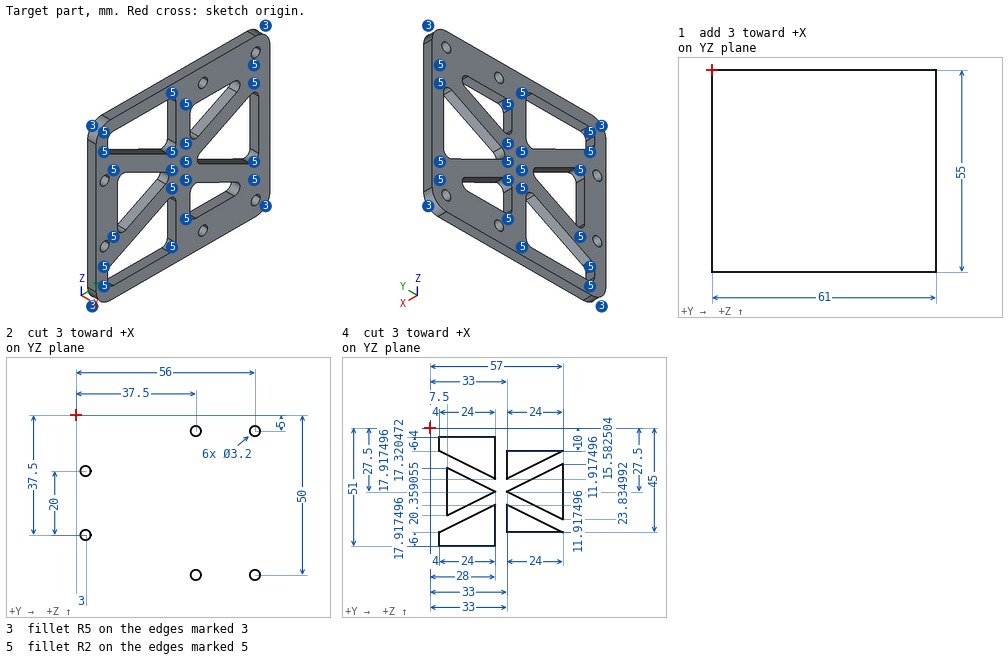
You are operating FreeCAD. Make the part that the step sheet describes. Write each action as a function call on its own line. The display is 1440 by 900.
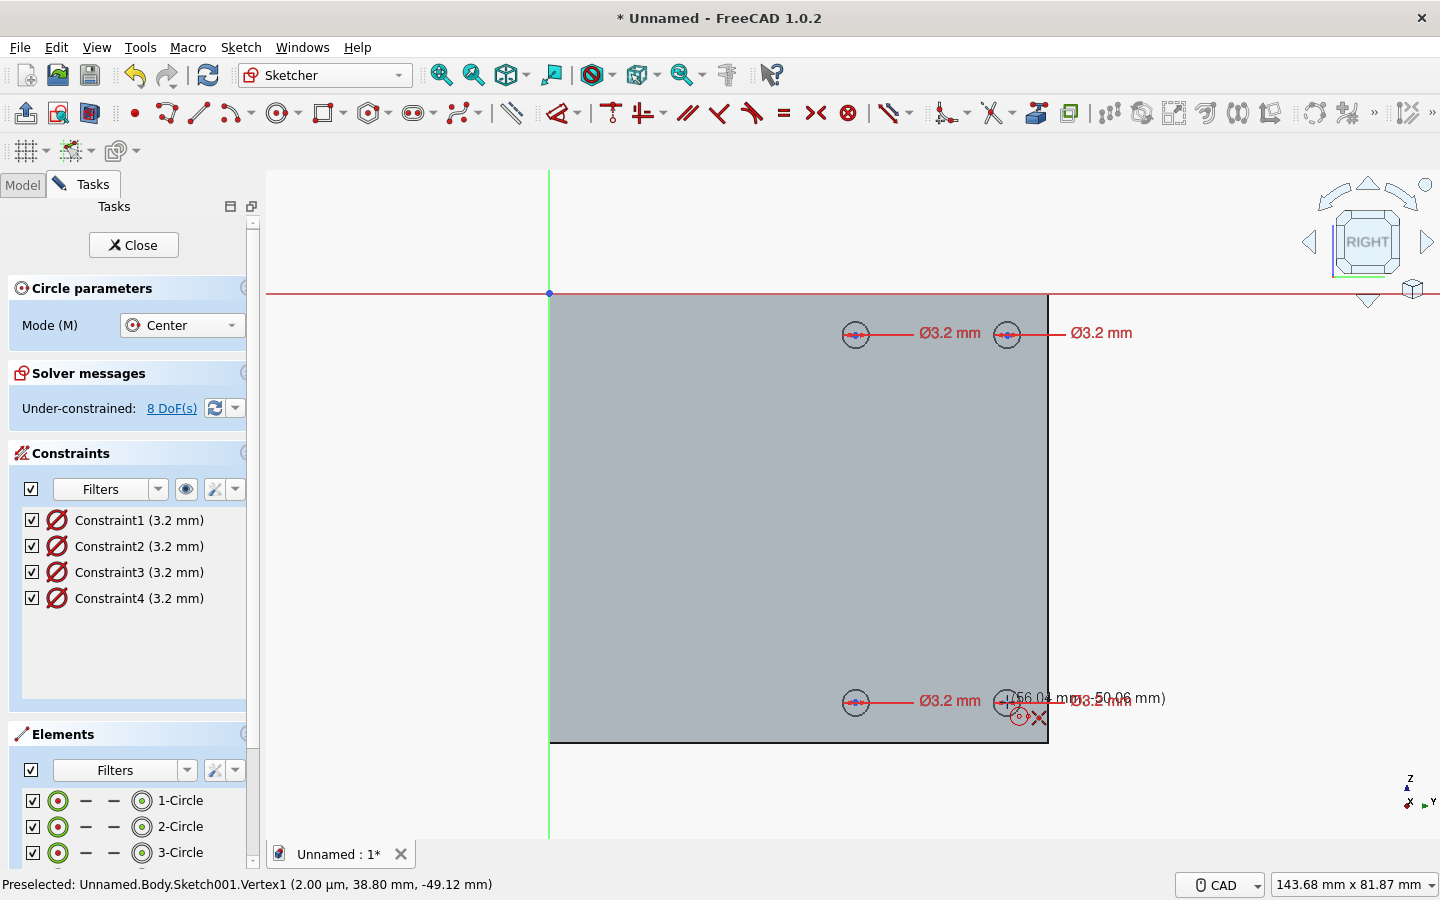
scroll(574, 600, up, 3)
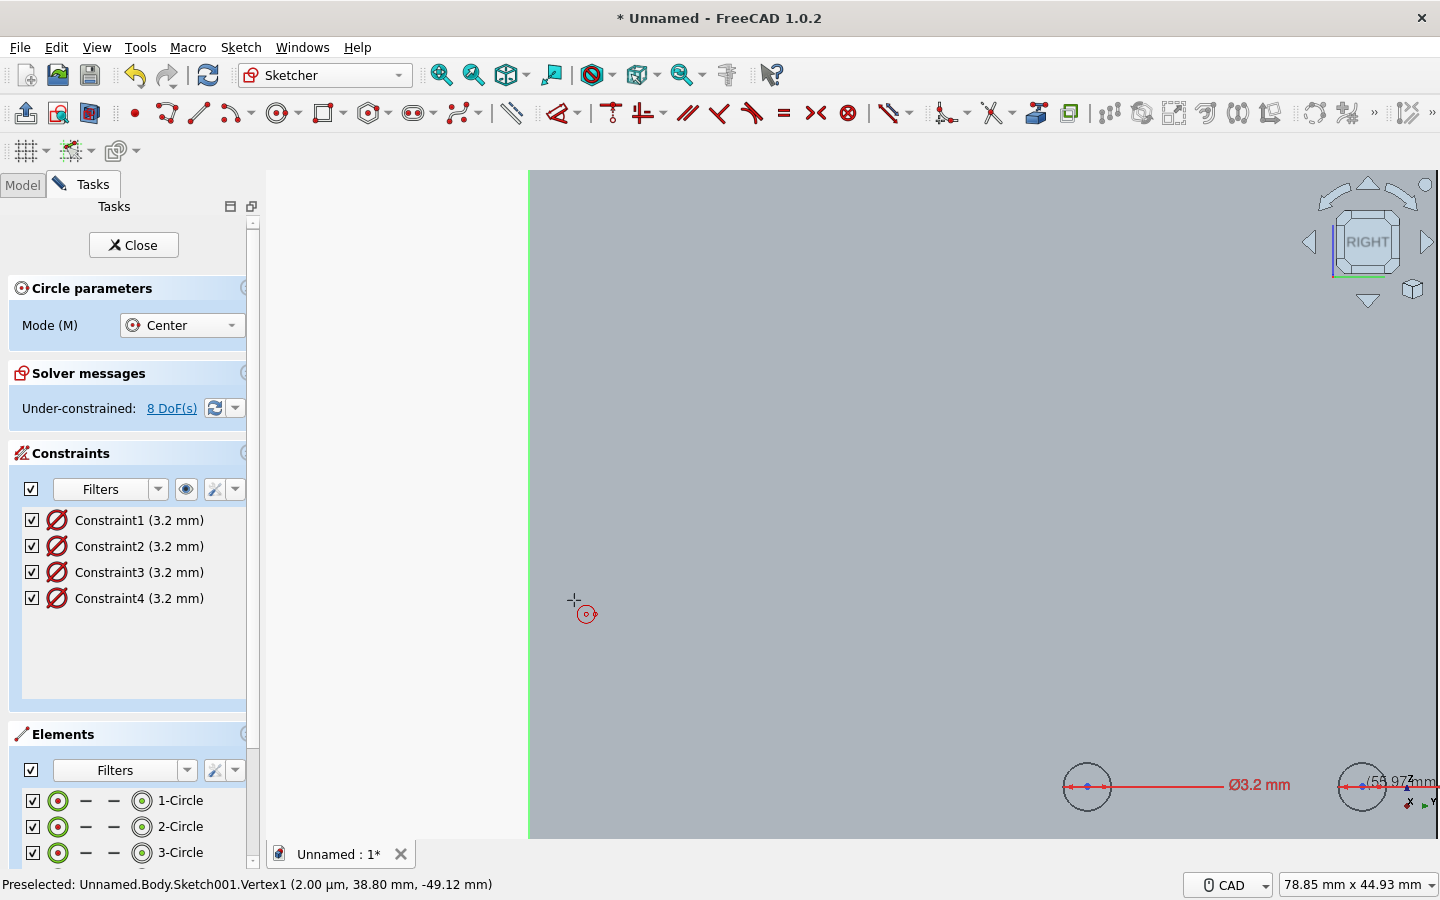
click(574, 600)
move(590, 583)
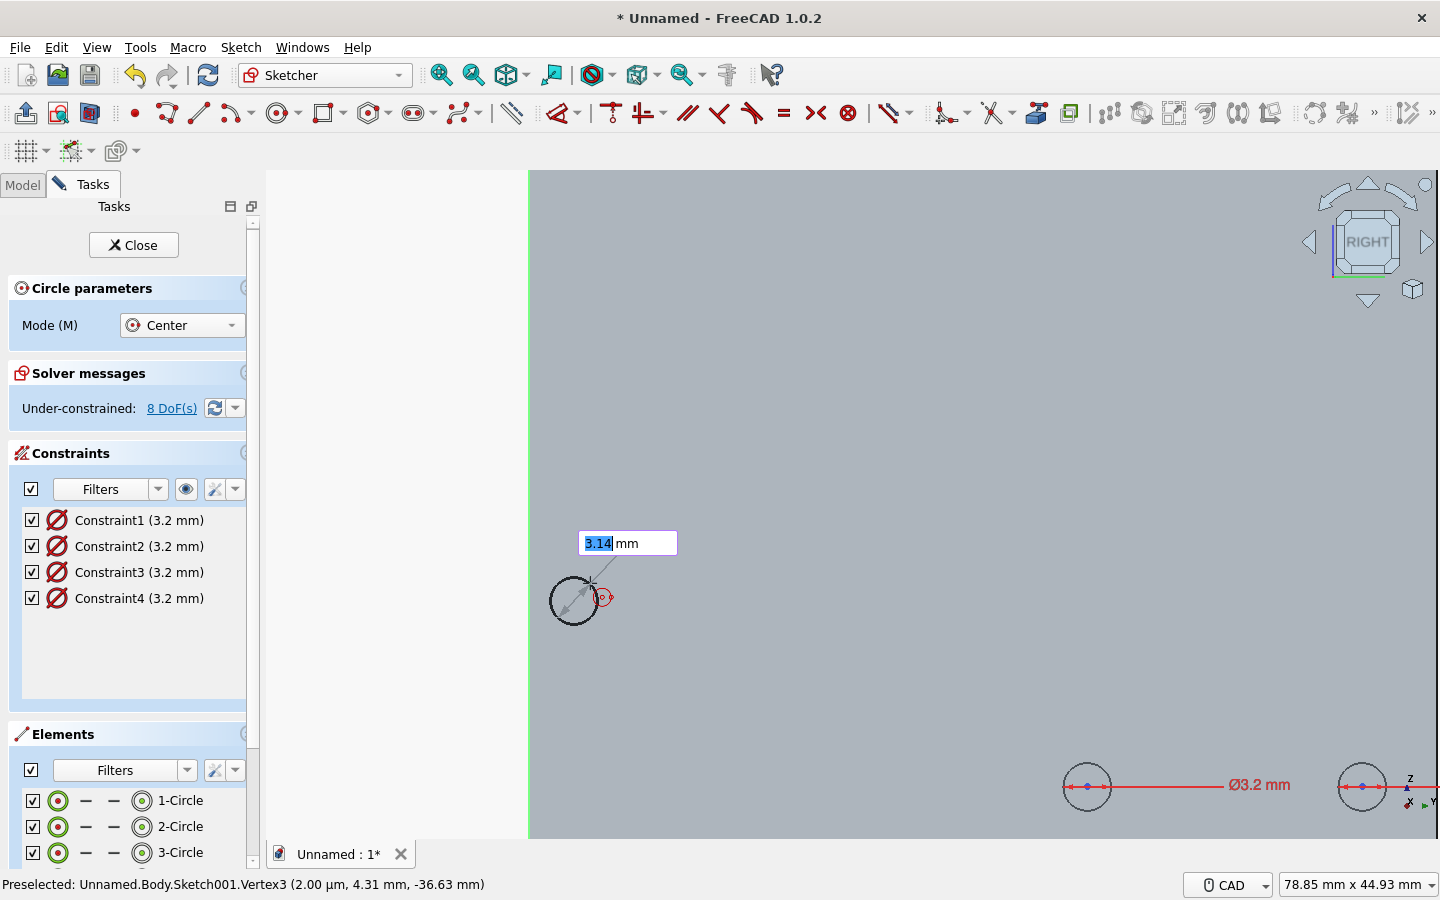
text(3.2)
key(Return)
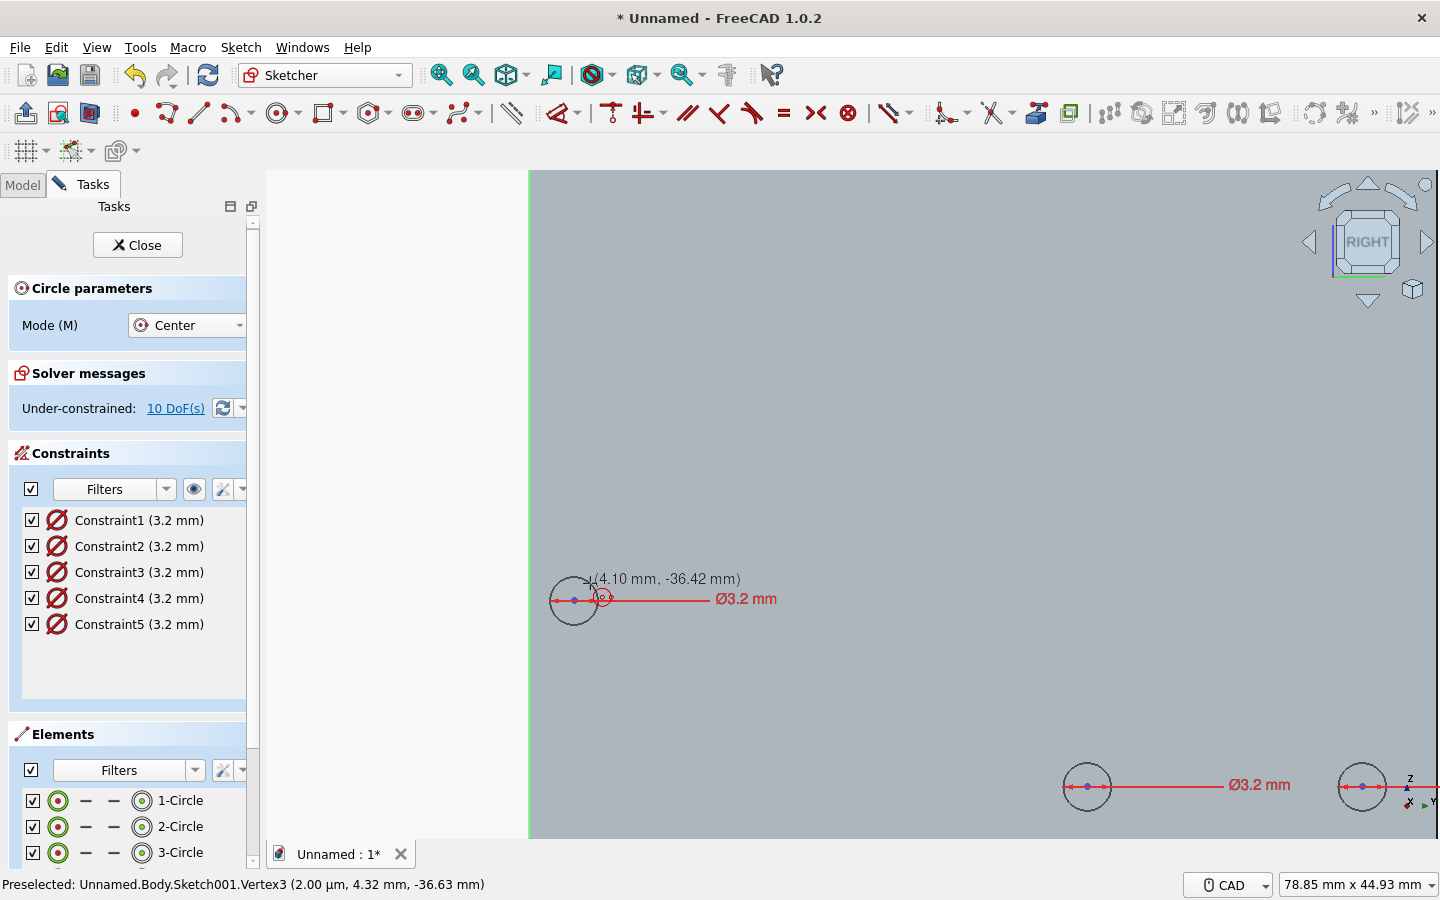
click(574, 302)
move(590, 285)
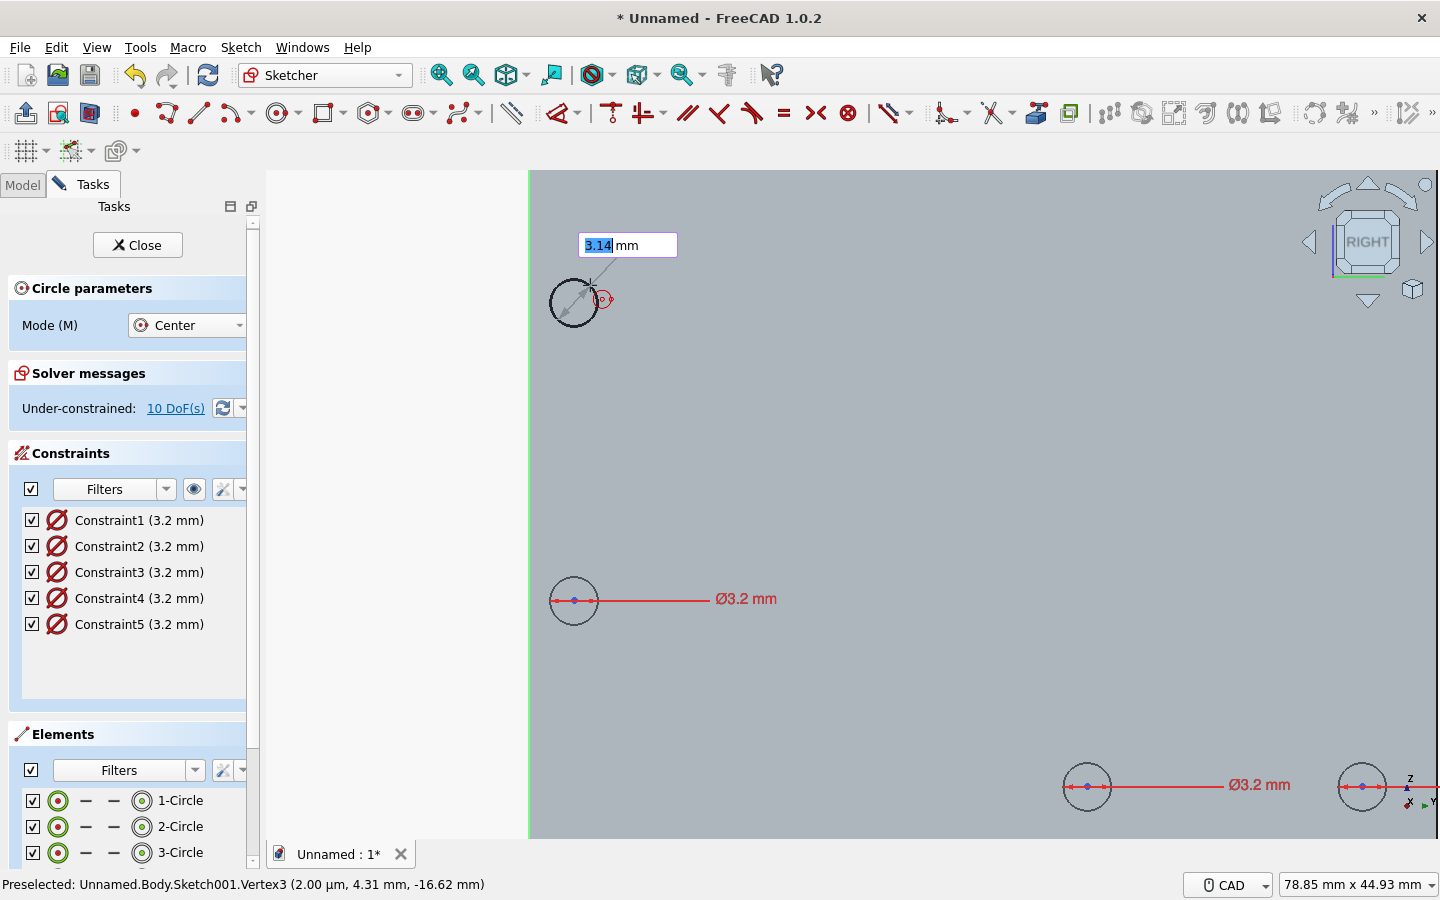
text(3.2)
key(Return)
key(Escape)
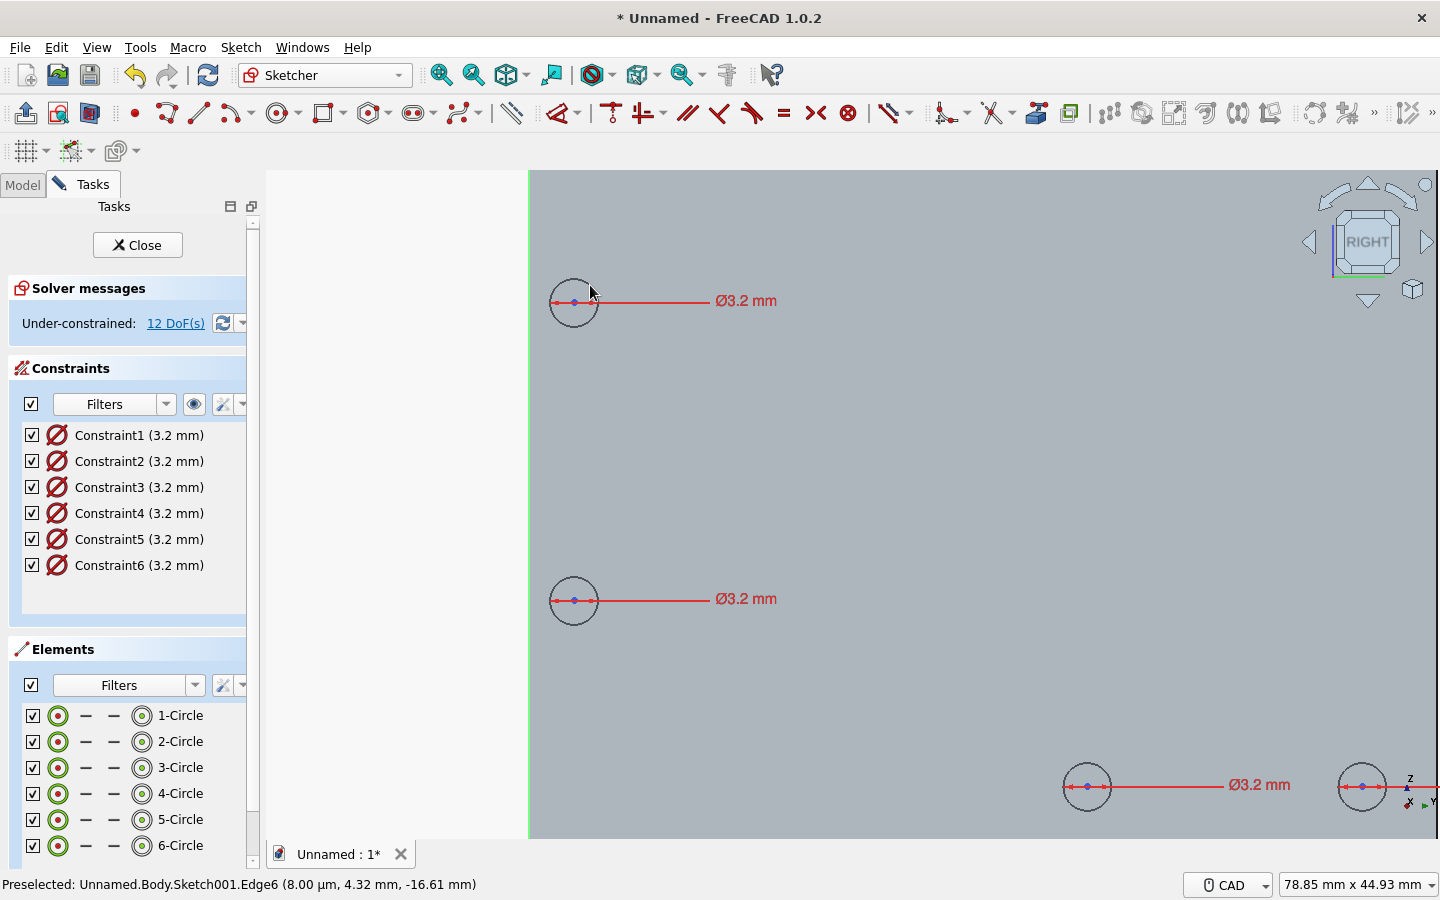
scroll(574, 600, down, 3)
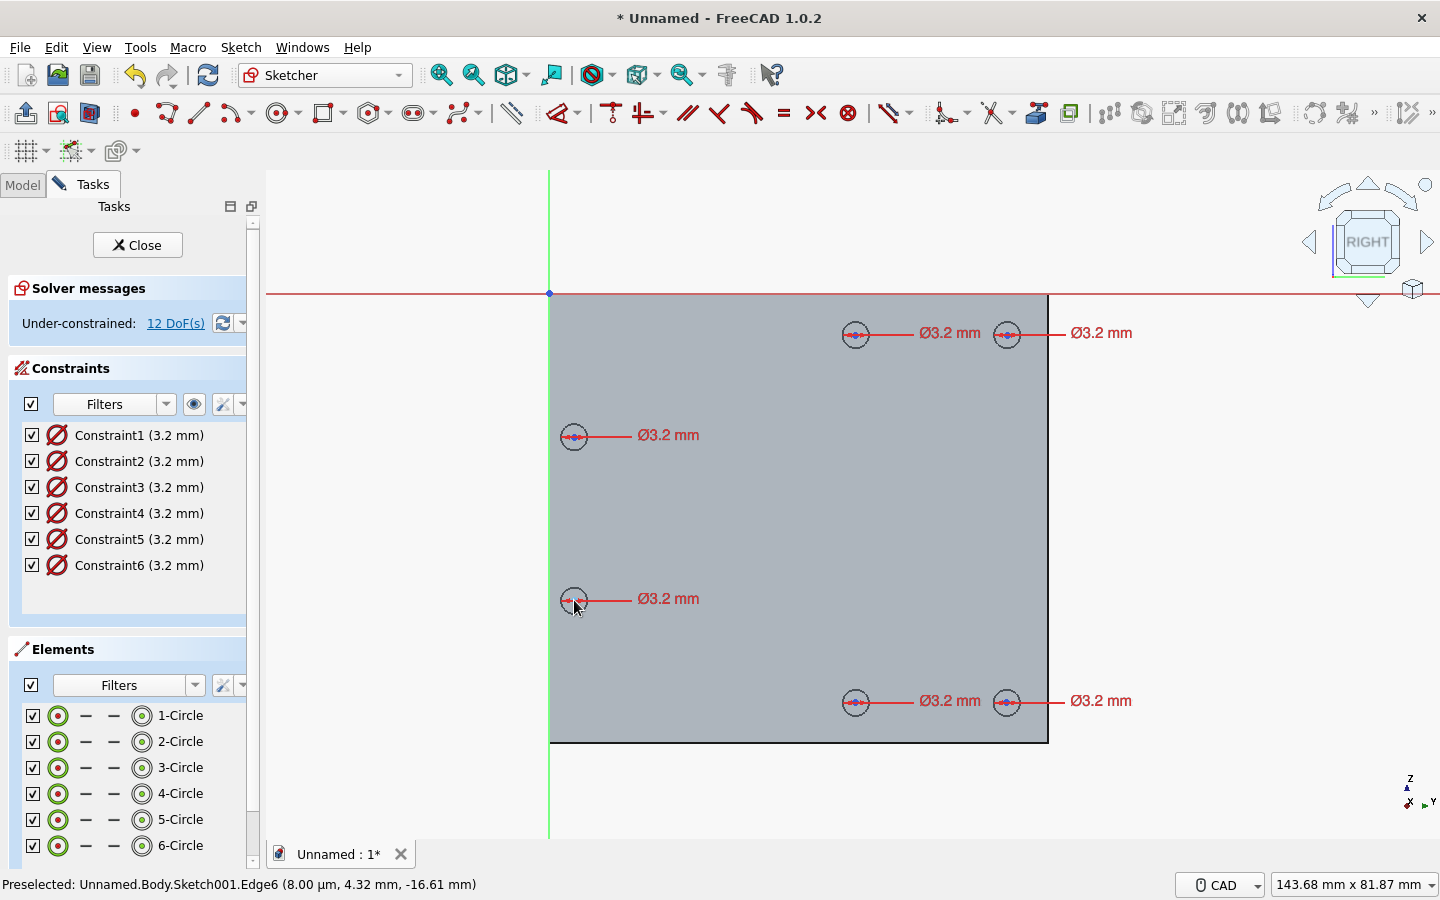
click(1007, 335)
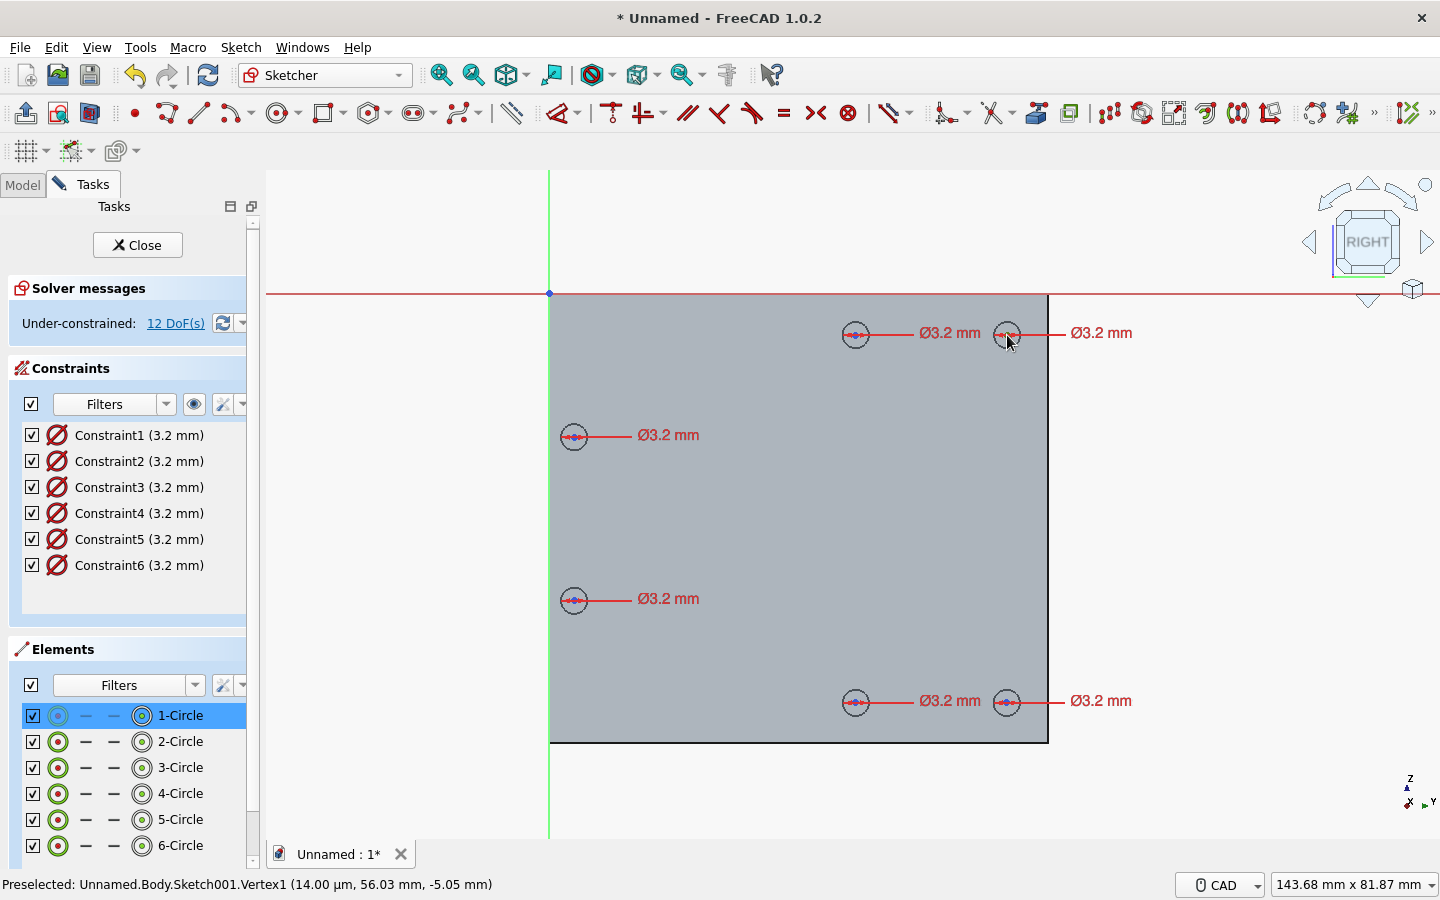
click(856, 335)